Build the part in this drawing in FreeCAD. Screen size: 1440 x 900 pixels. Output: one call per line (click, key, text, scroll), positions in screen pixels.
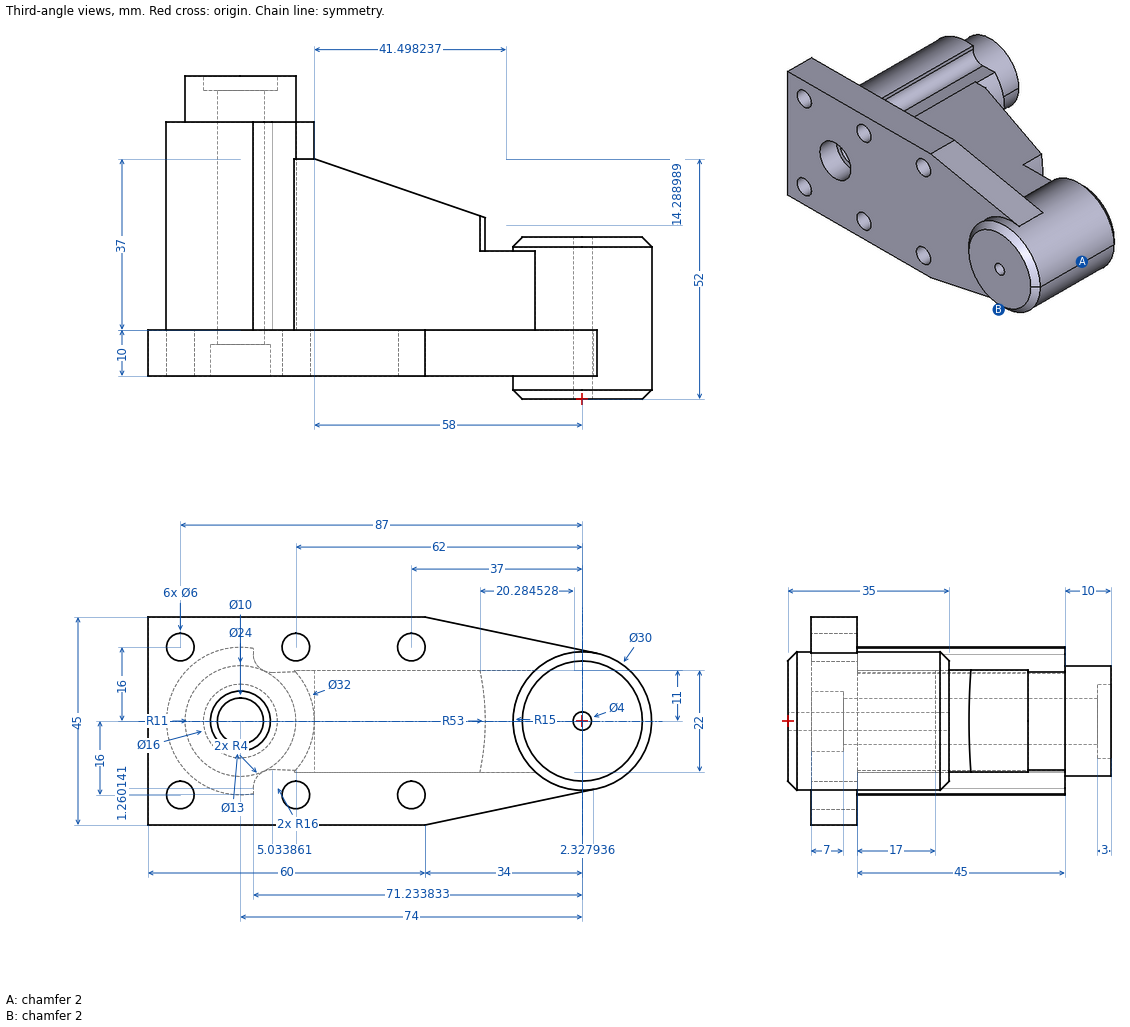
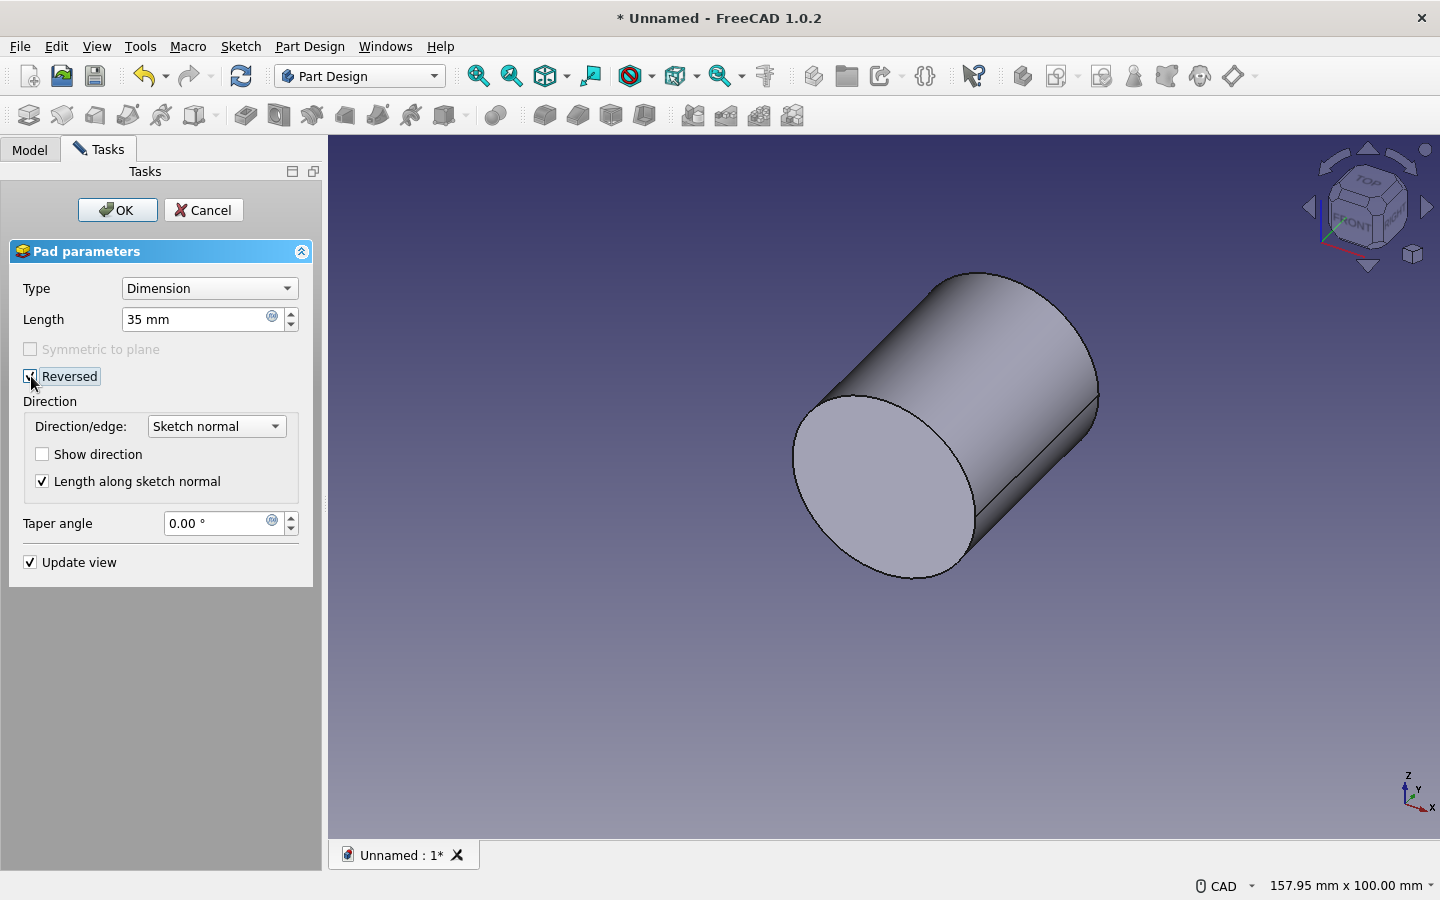
click(118, 210)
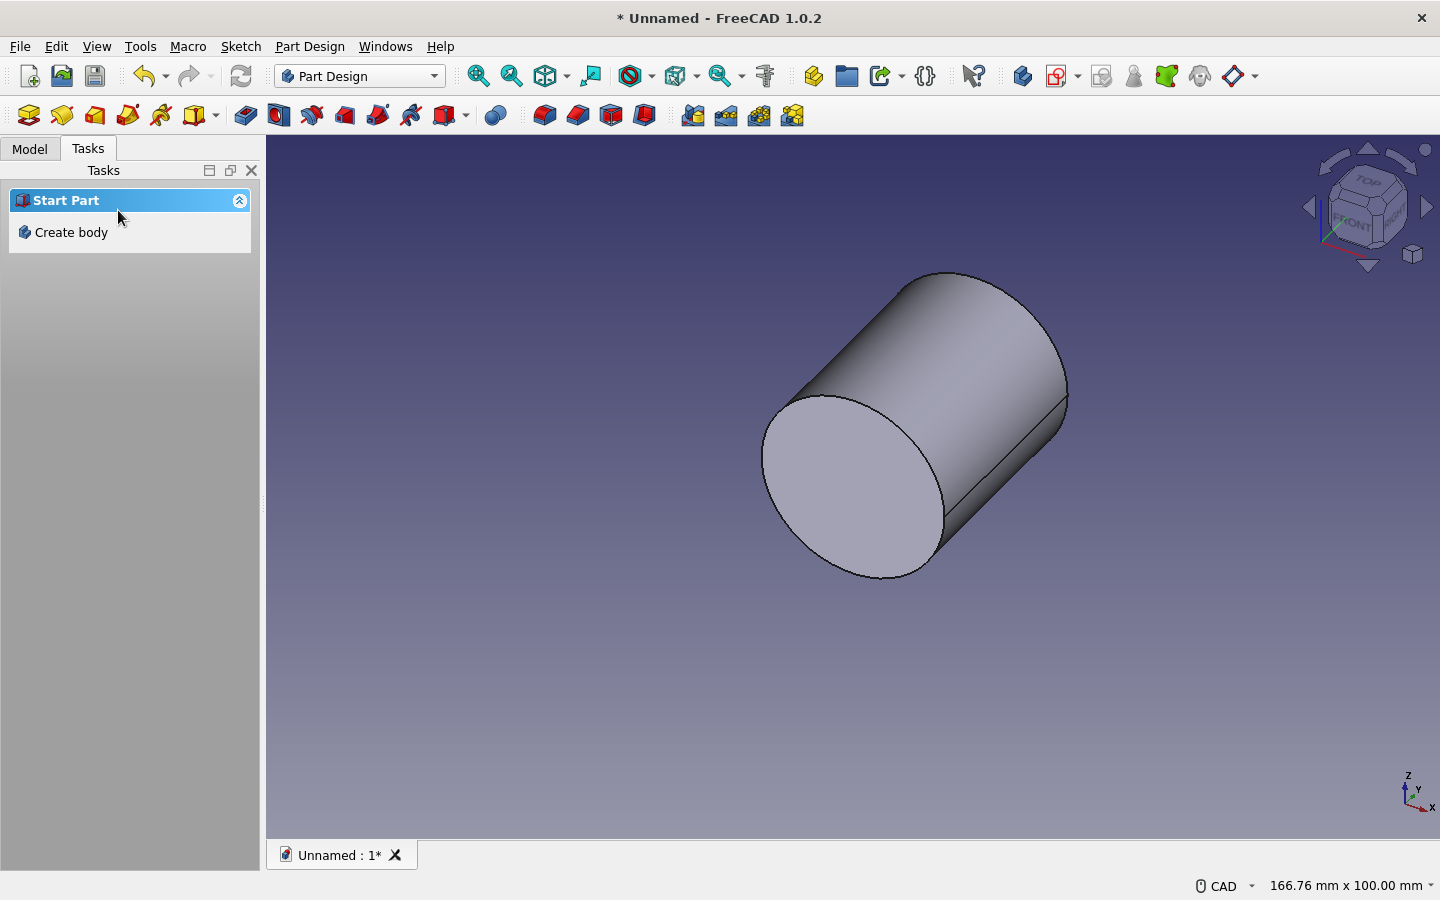
click(30, 148)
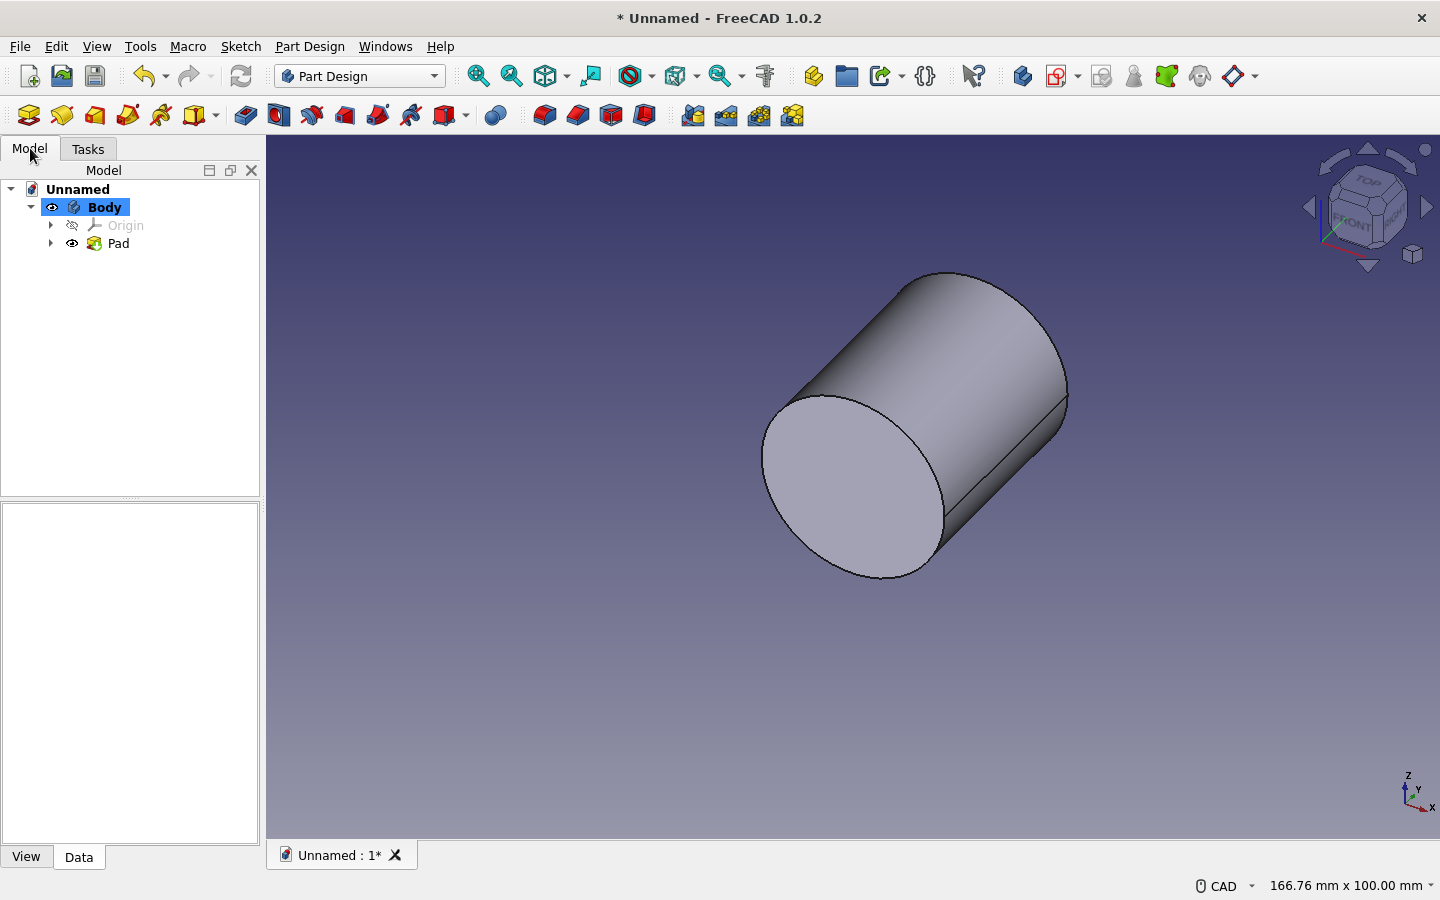
click(51, 225)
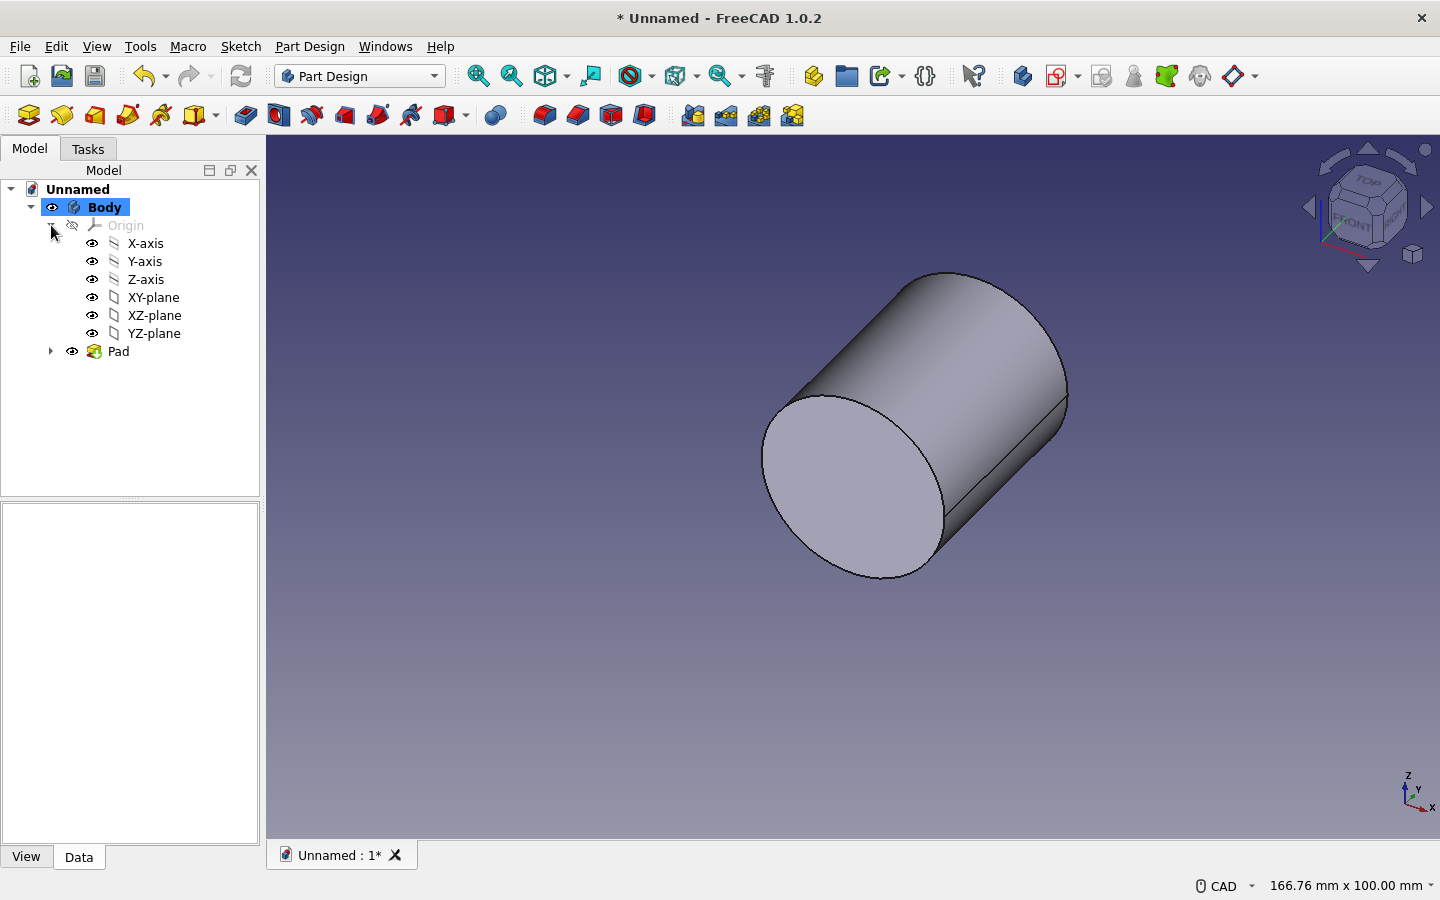
click(137, 315)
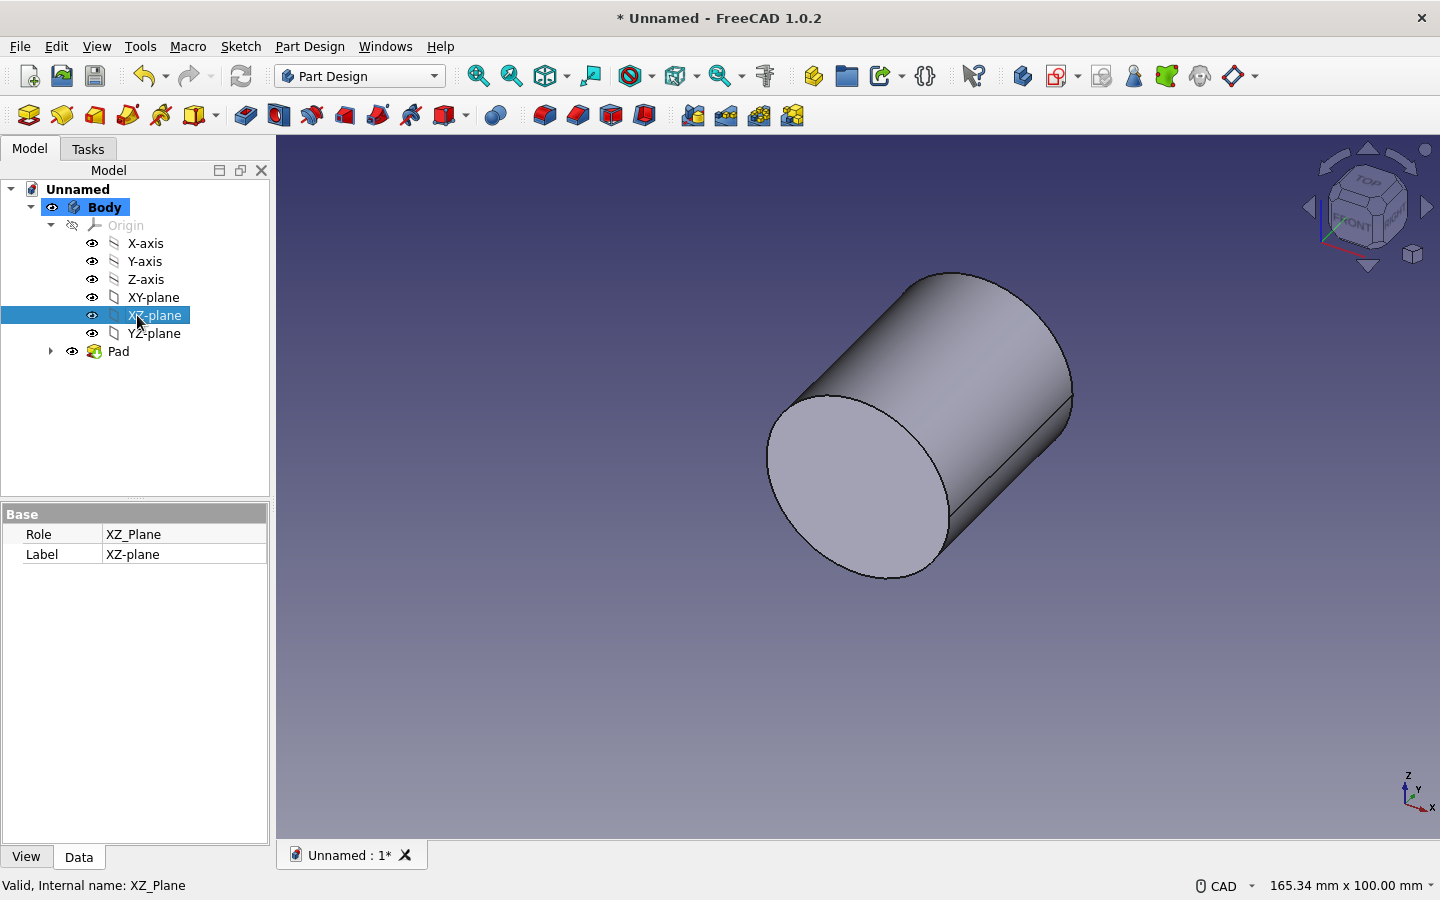
click(1232, 76)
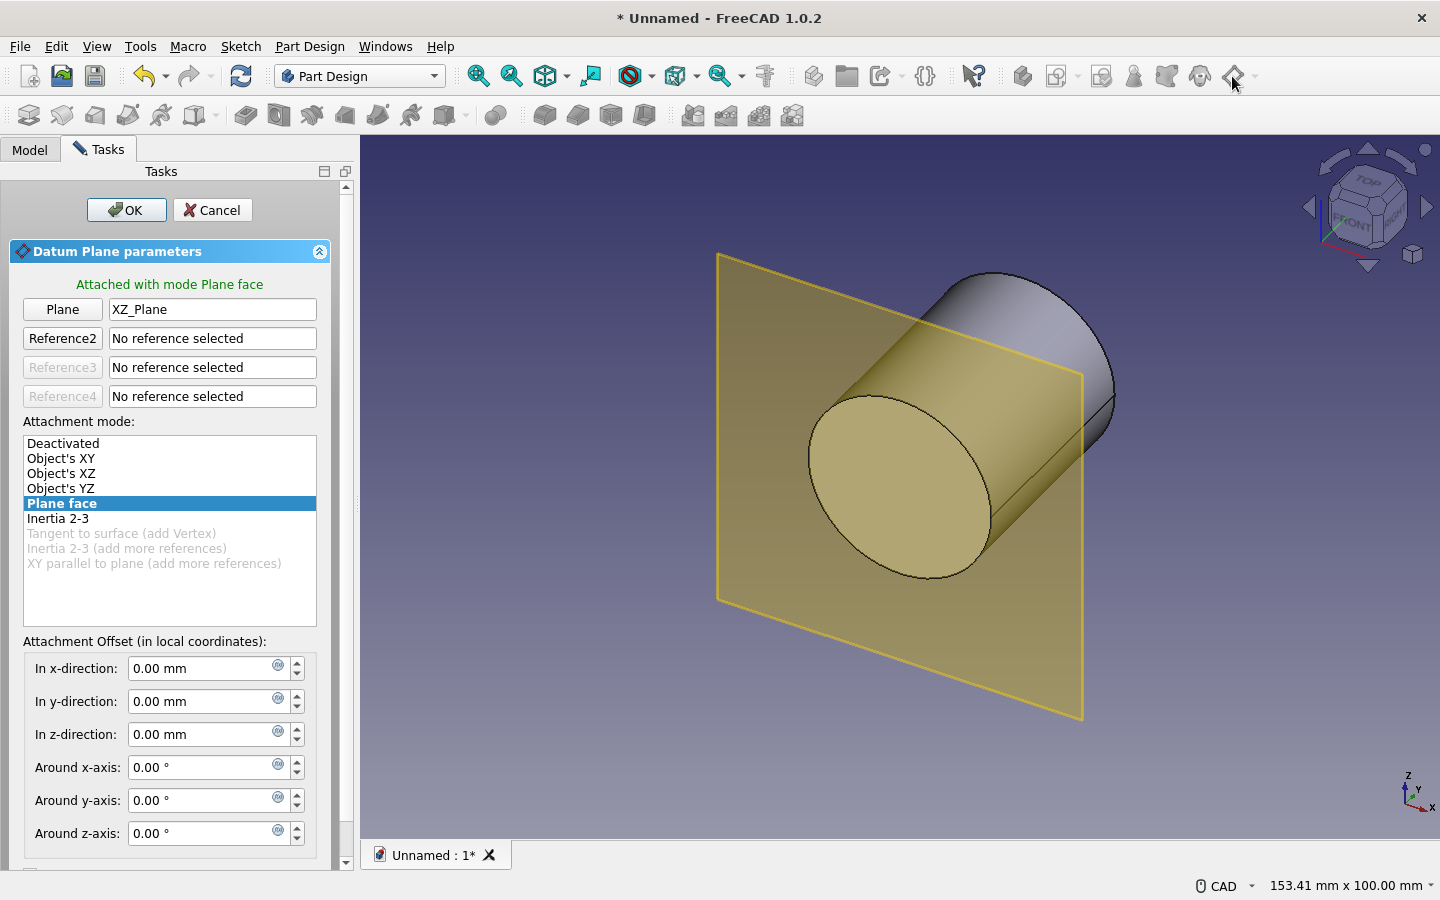
triple_click(210, 734)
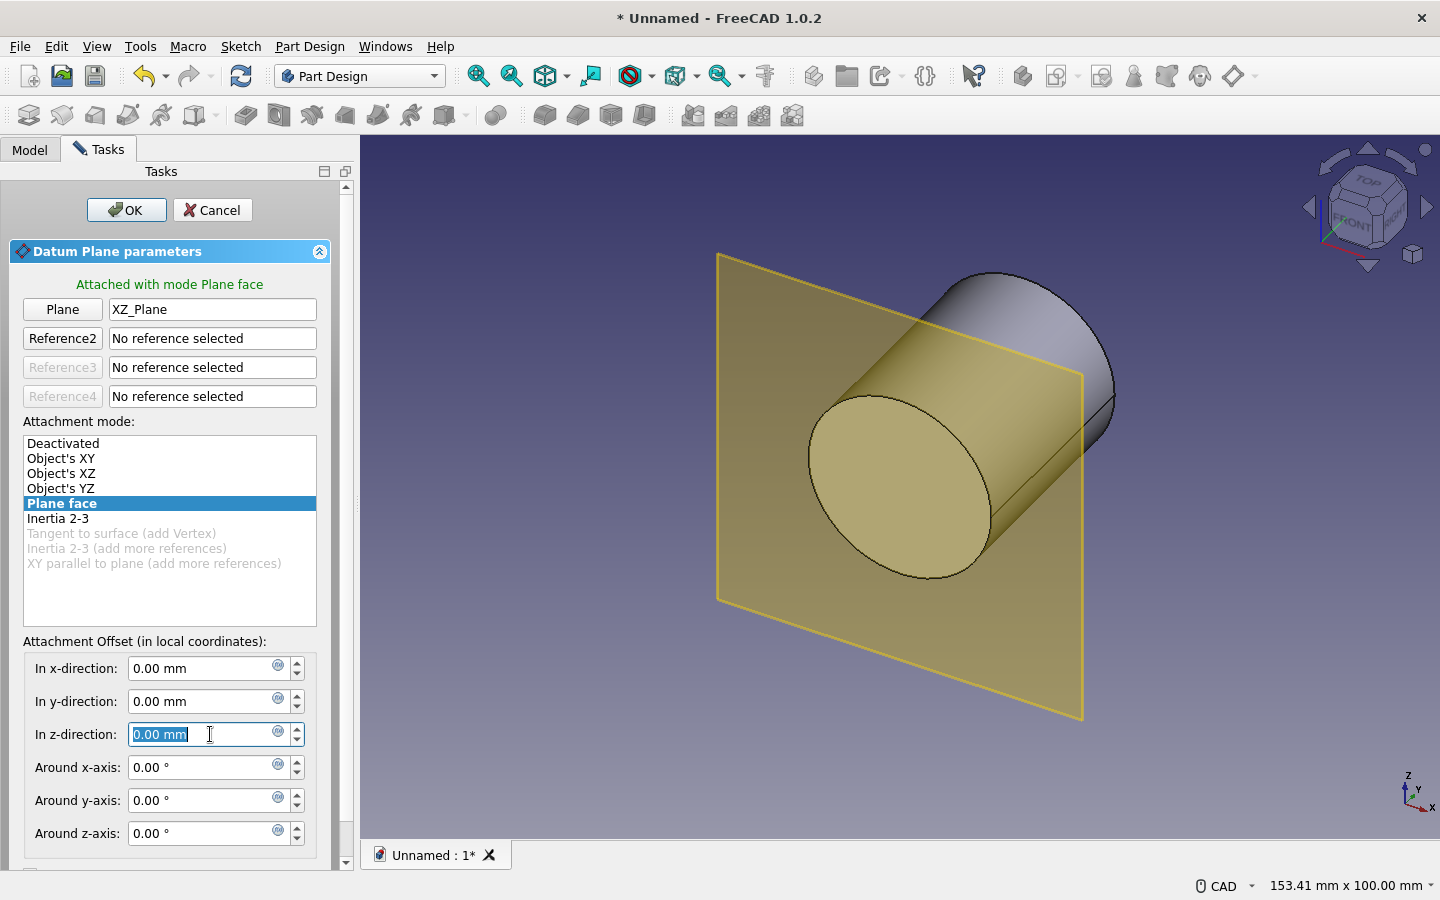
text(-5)
key(Tab)